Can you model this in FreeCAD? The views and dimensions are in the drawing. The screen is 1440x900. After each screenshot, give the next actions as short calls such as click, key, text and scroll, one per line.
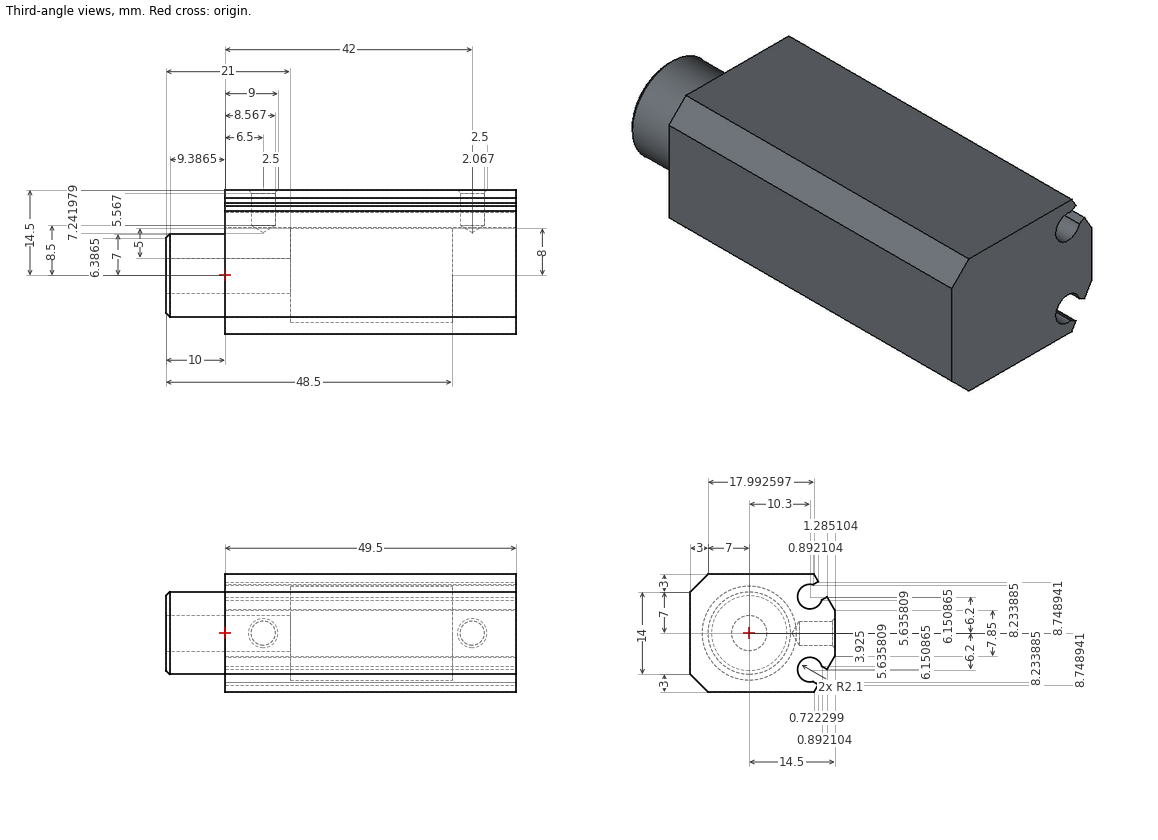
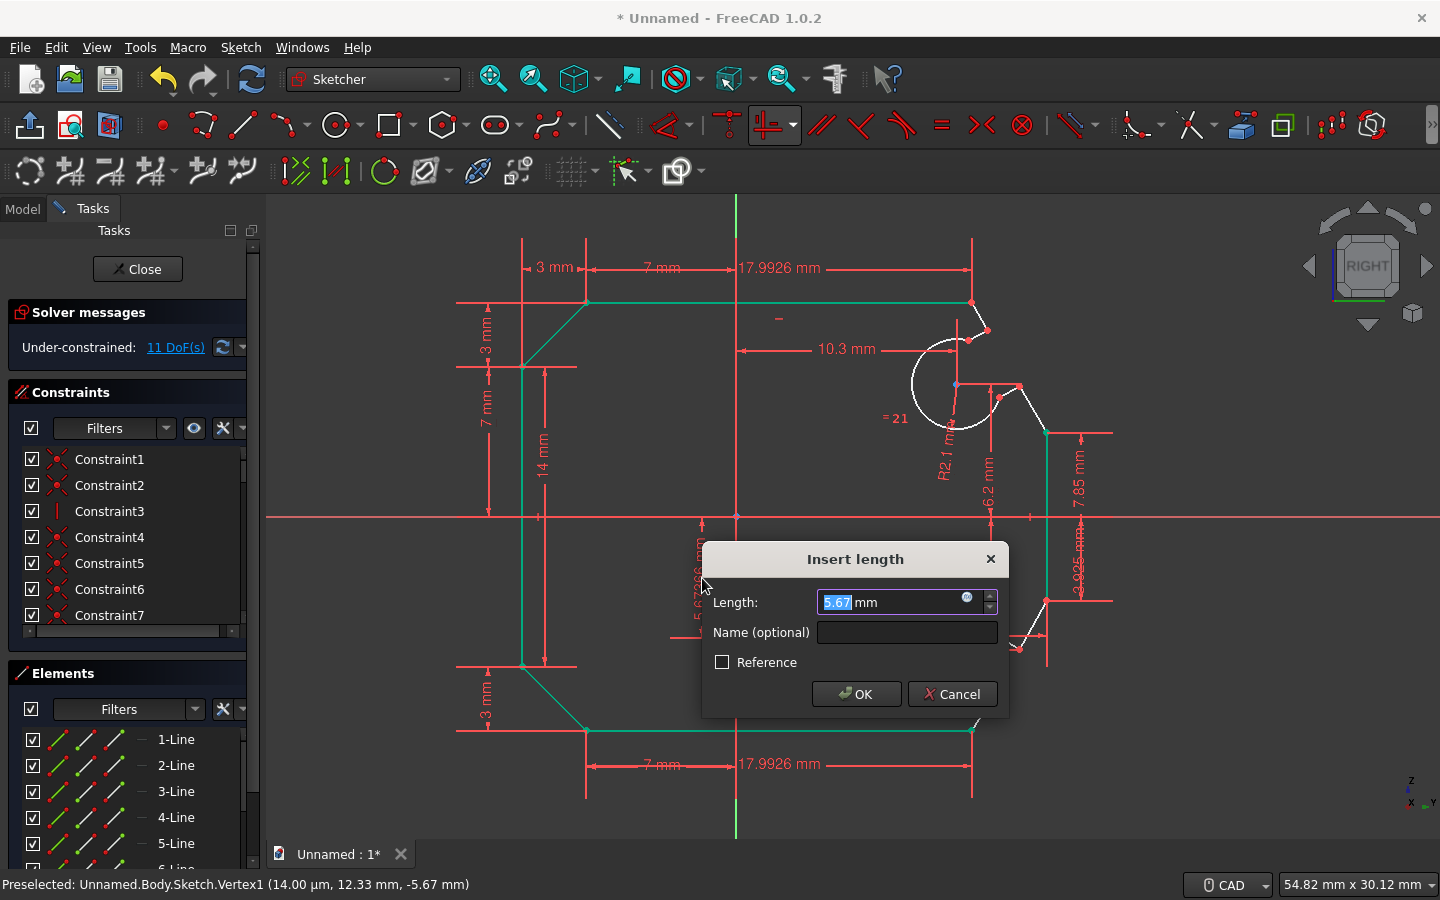
text(5.635809)
key(Return)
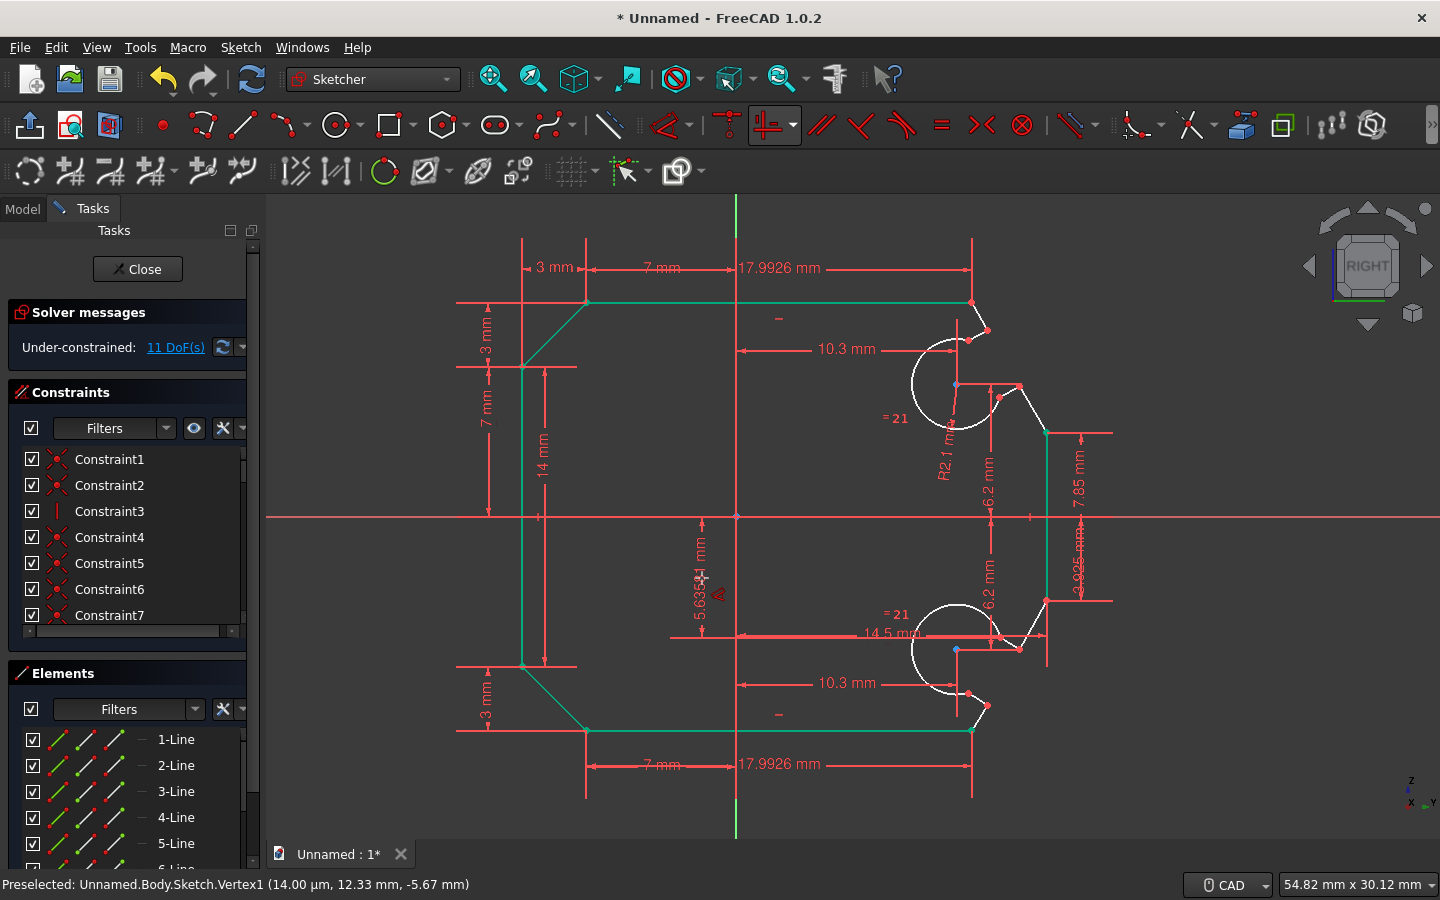
click(1020, 649)
click(1054, 629)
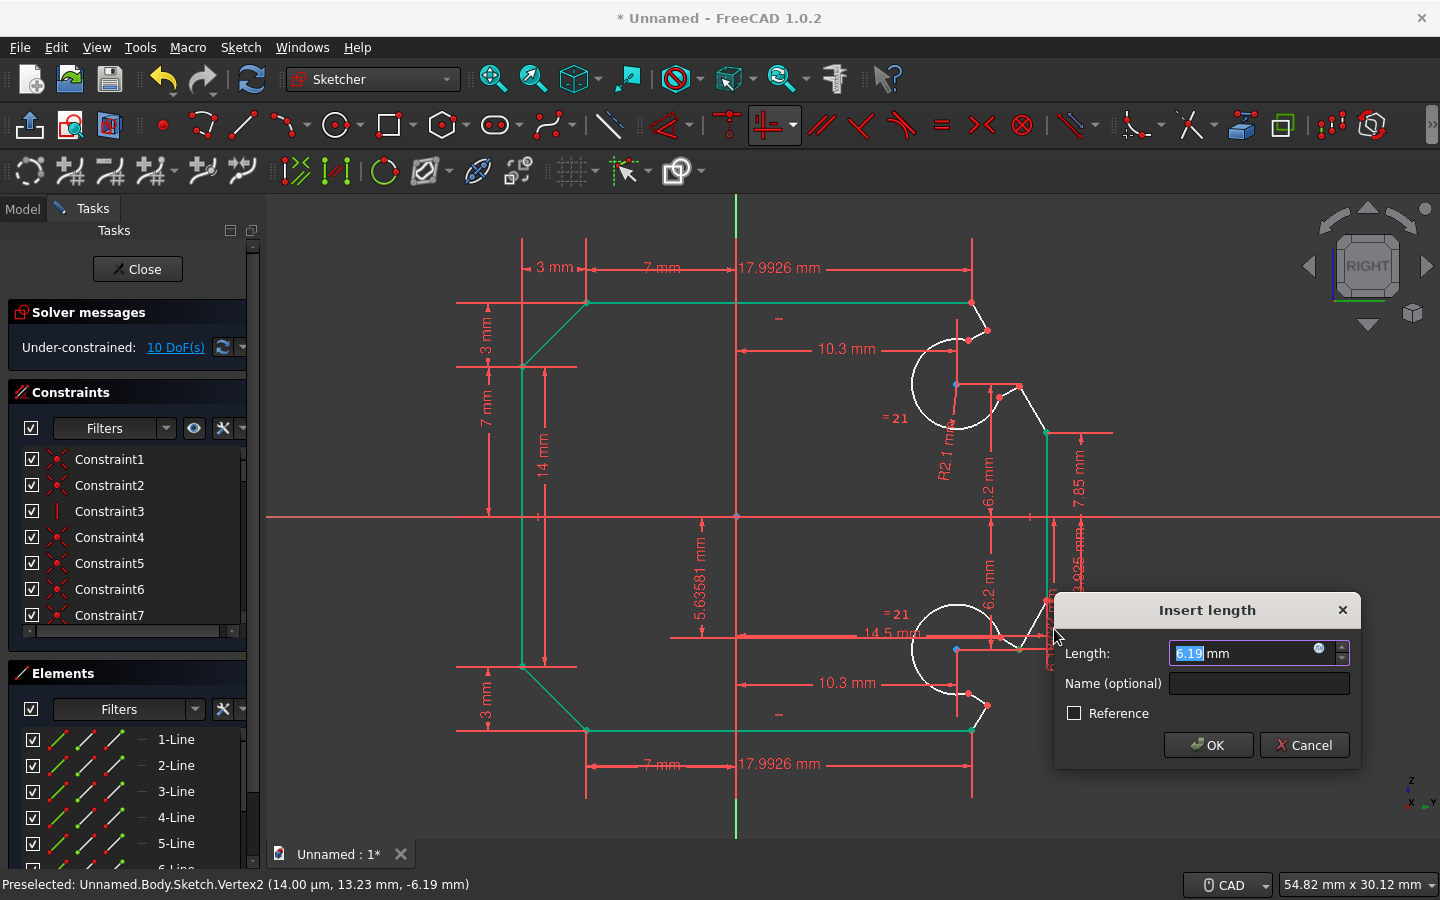
text(6.150865)
key(Return)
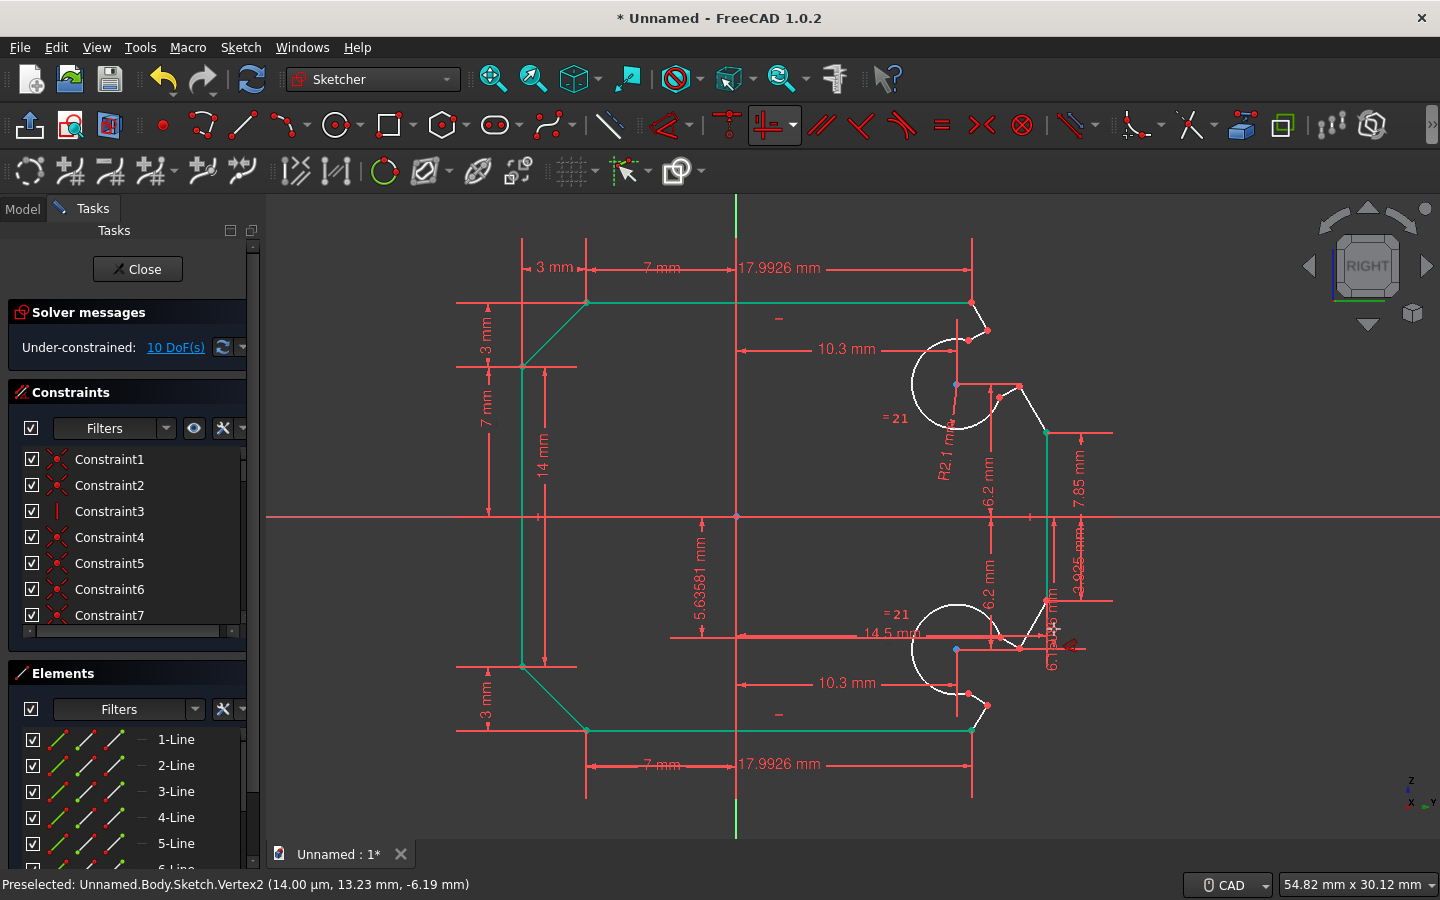
click(1020, 386)
click(1054, 406)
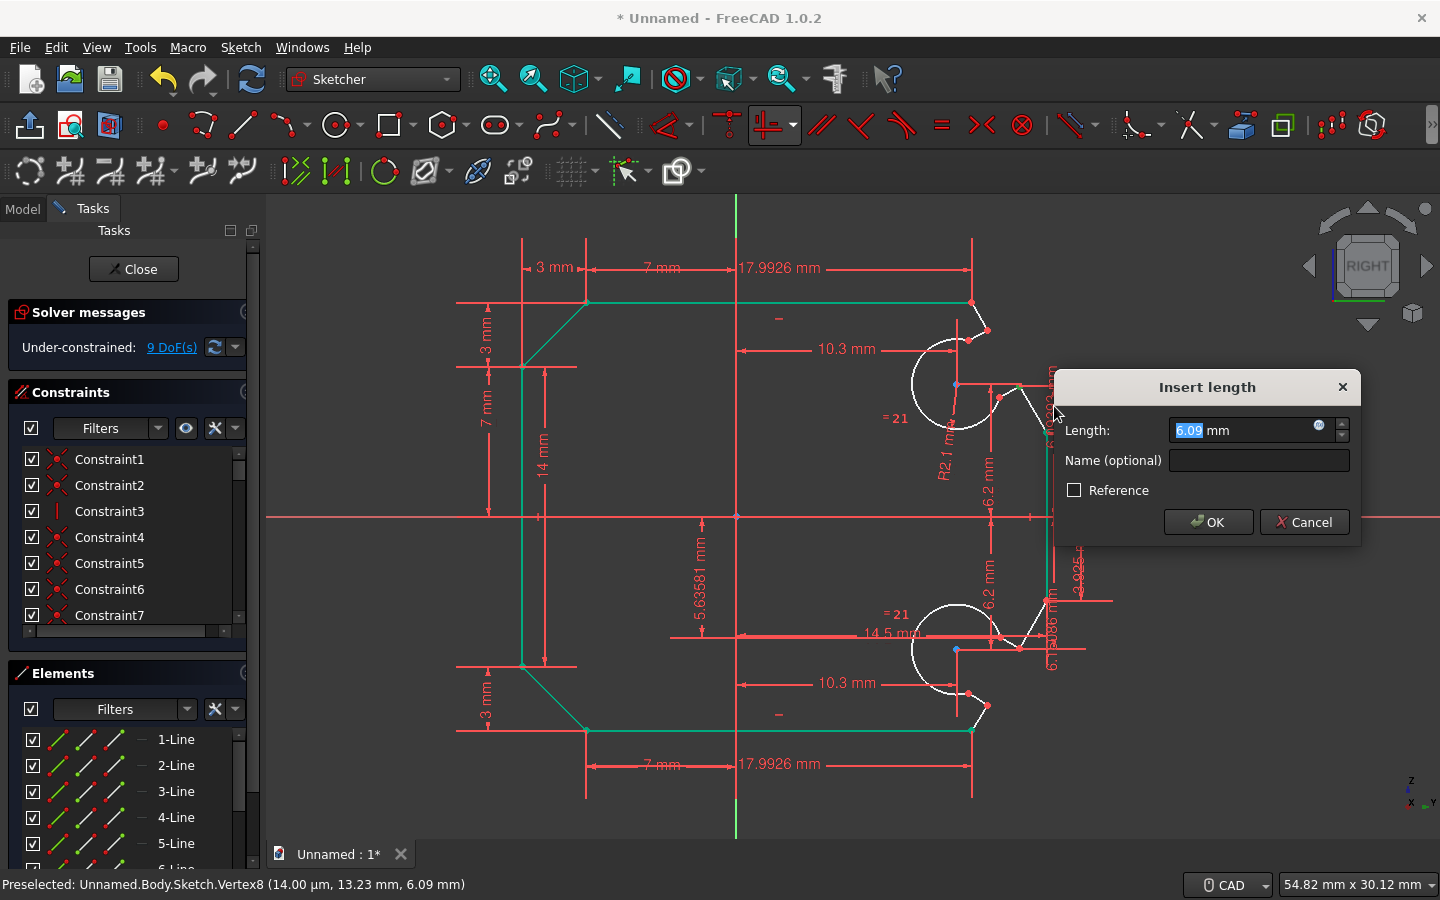
text(6.150865)
key(Return)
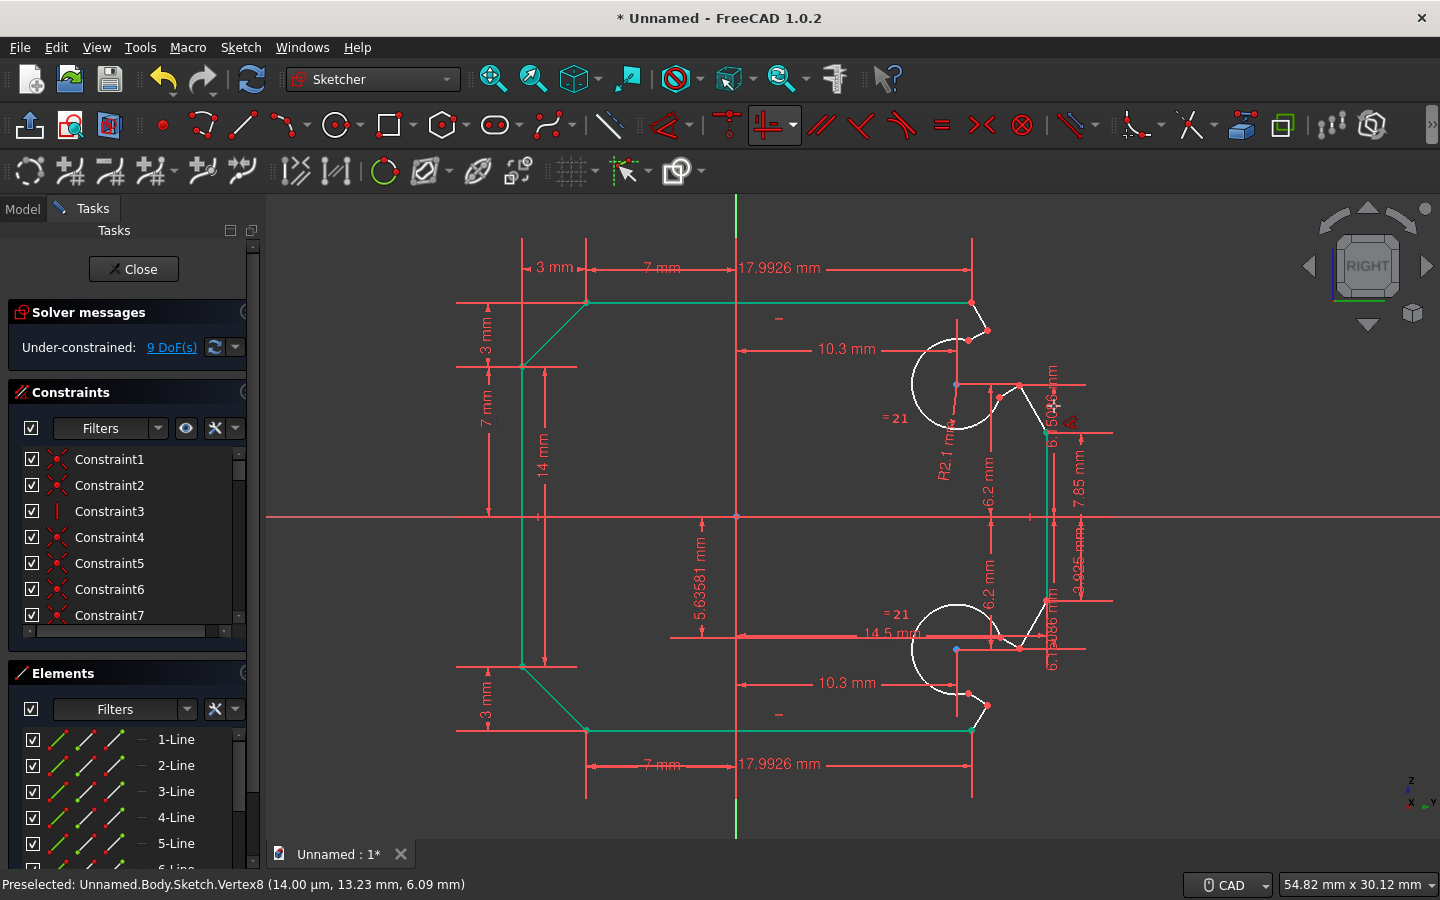
click(1000, 397)
click(702, 457)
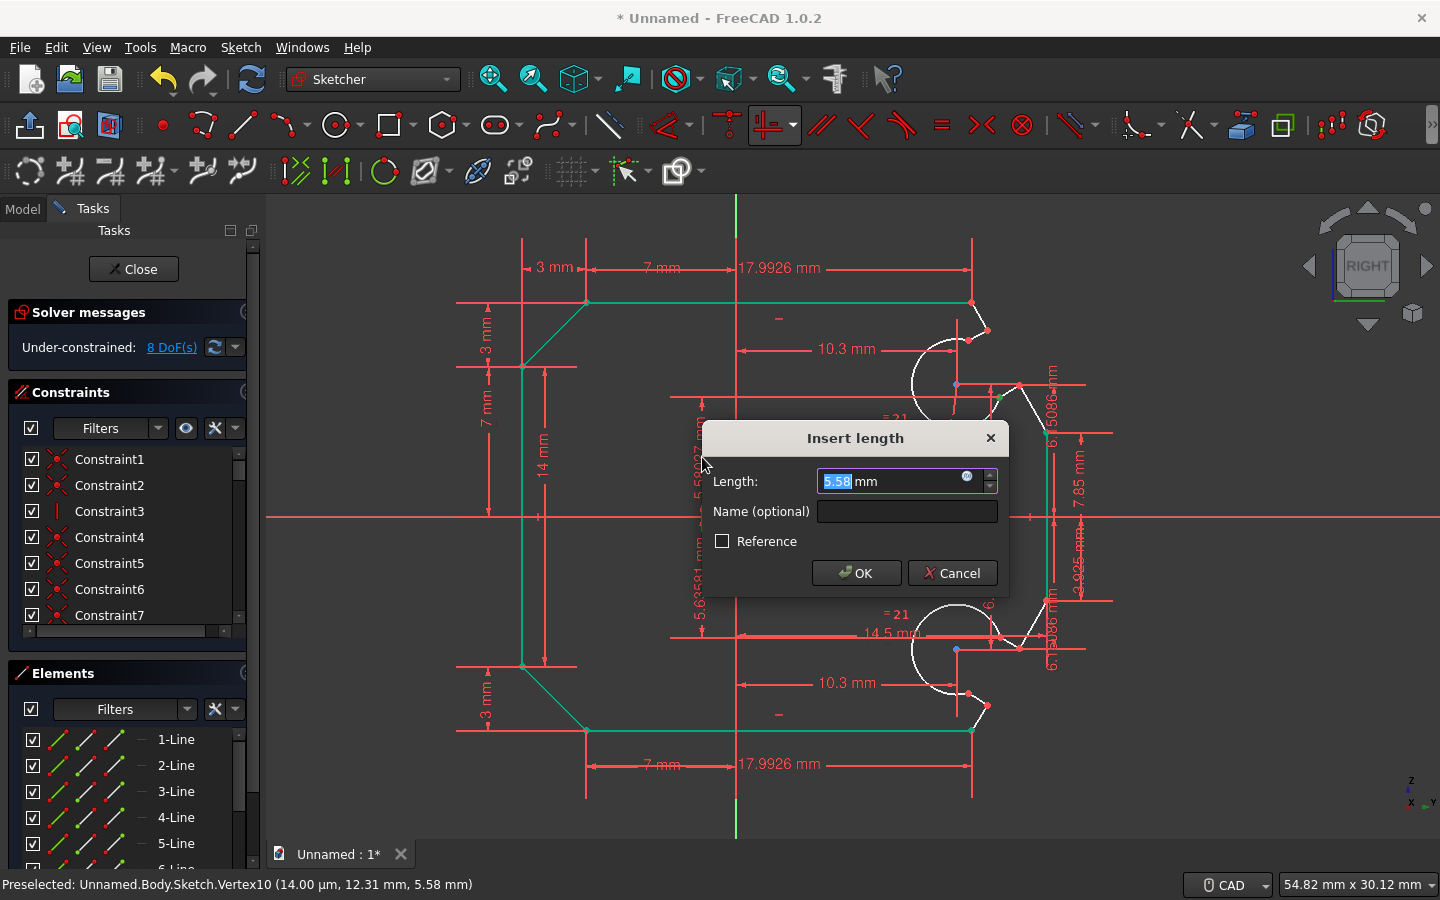
text(5.635809)
key(Return)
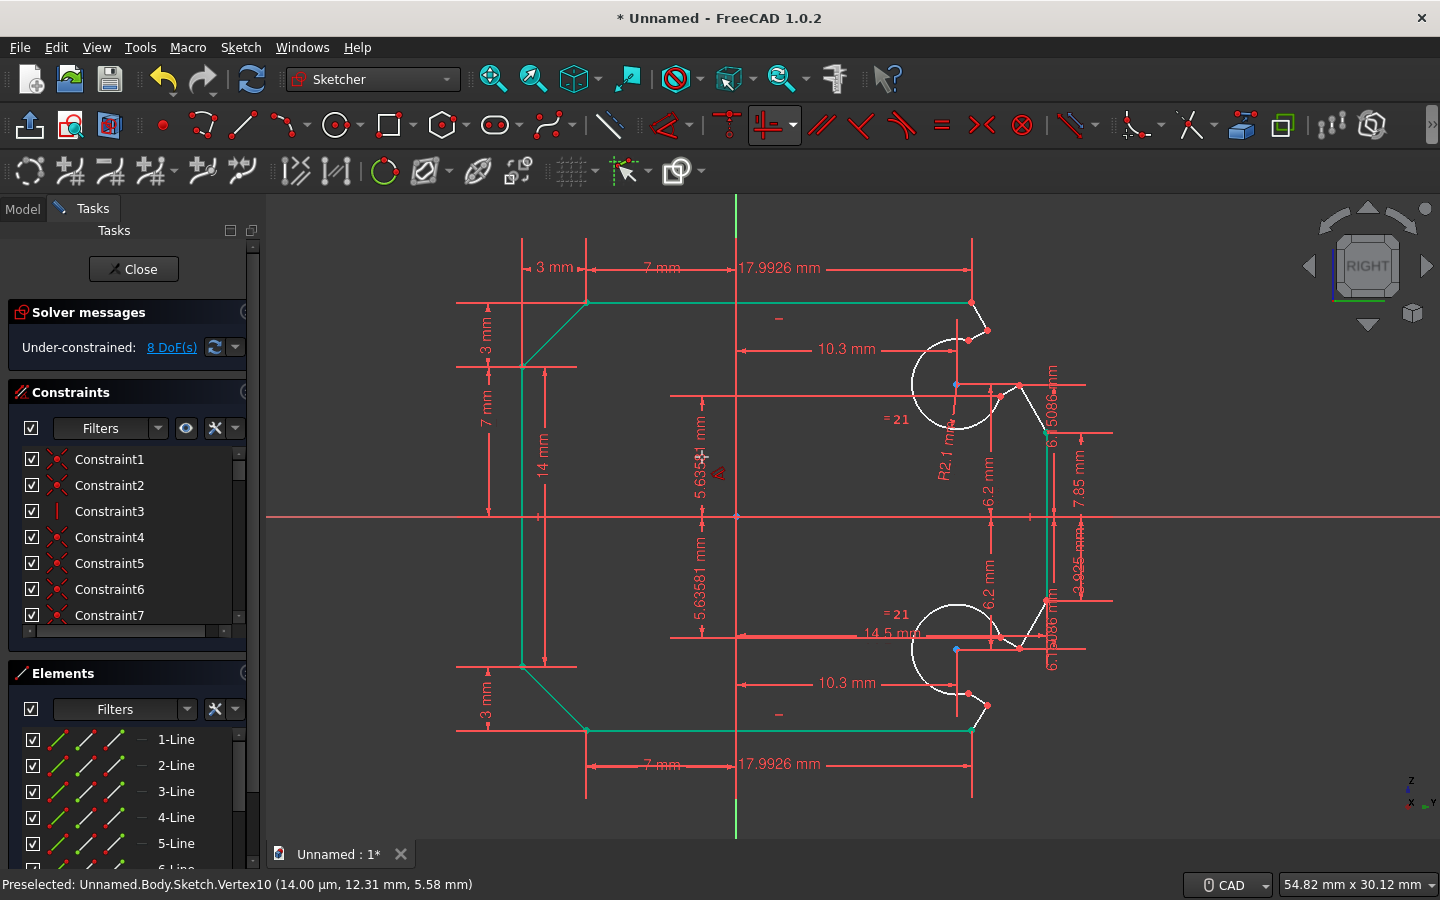
click(969, 341)
click(1003, 429)